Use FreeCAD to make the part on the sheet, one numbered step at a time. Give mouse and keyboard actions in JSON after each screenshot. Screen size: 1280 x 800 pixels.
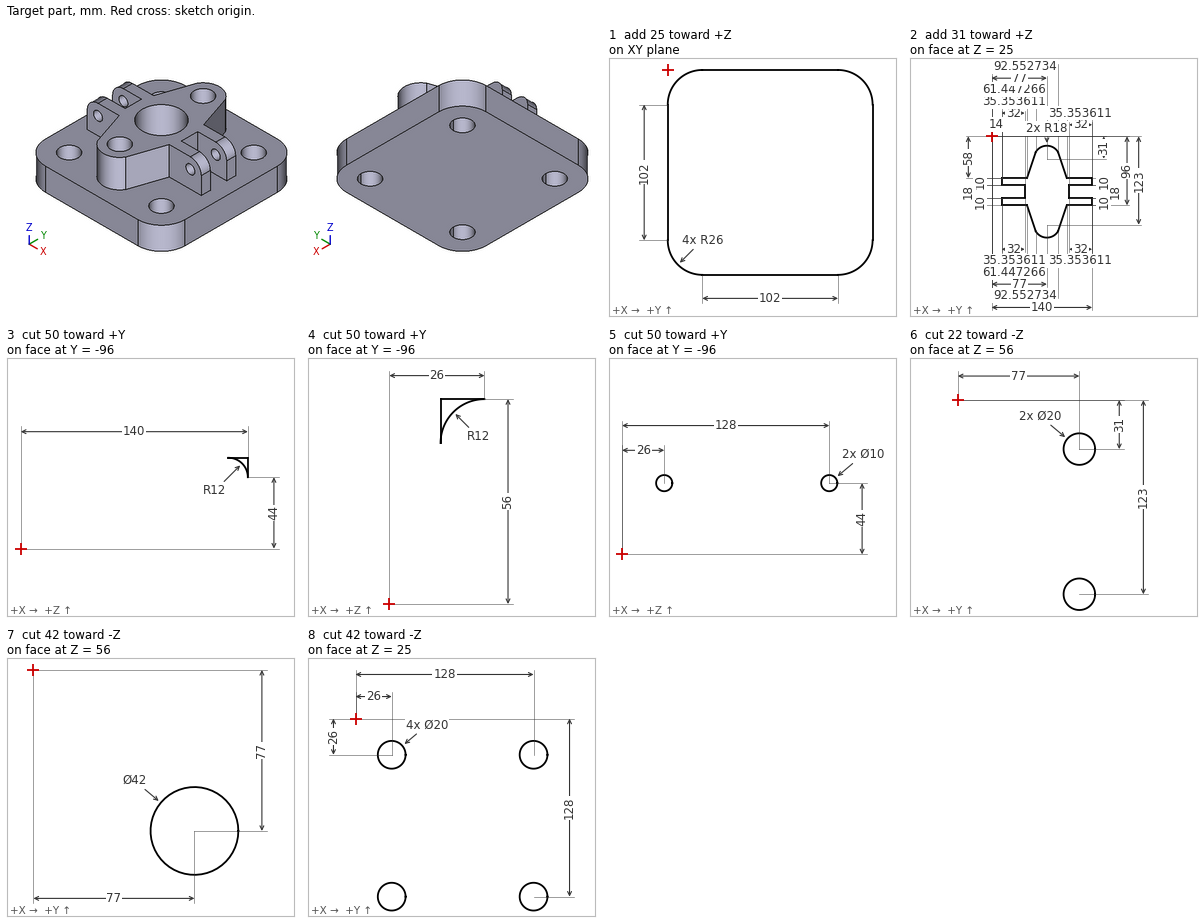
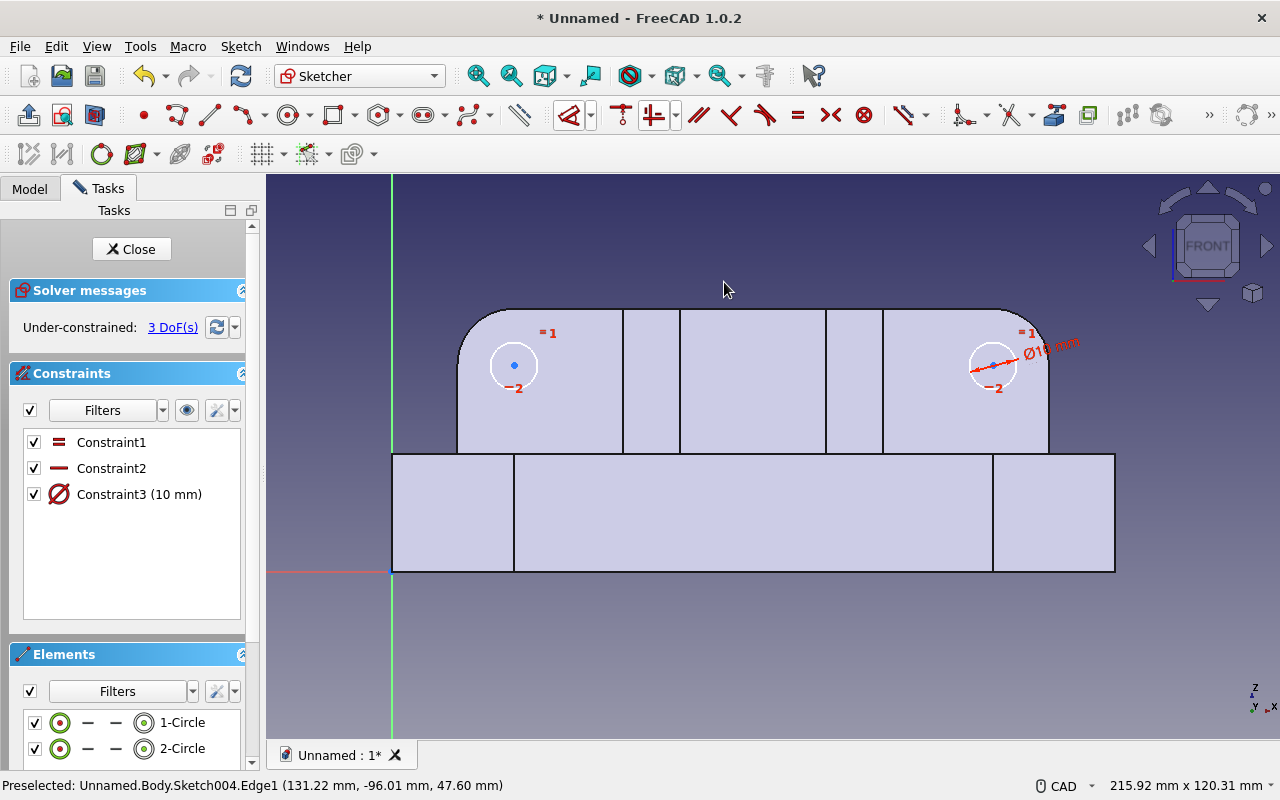
{"action": "left_click", "coordinate": [993, 366]}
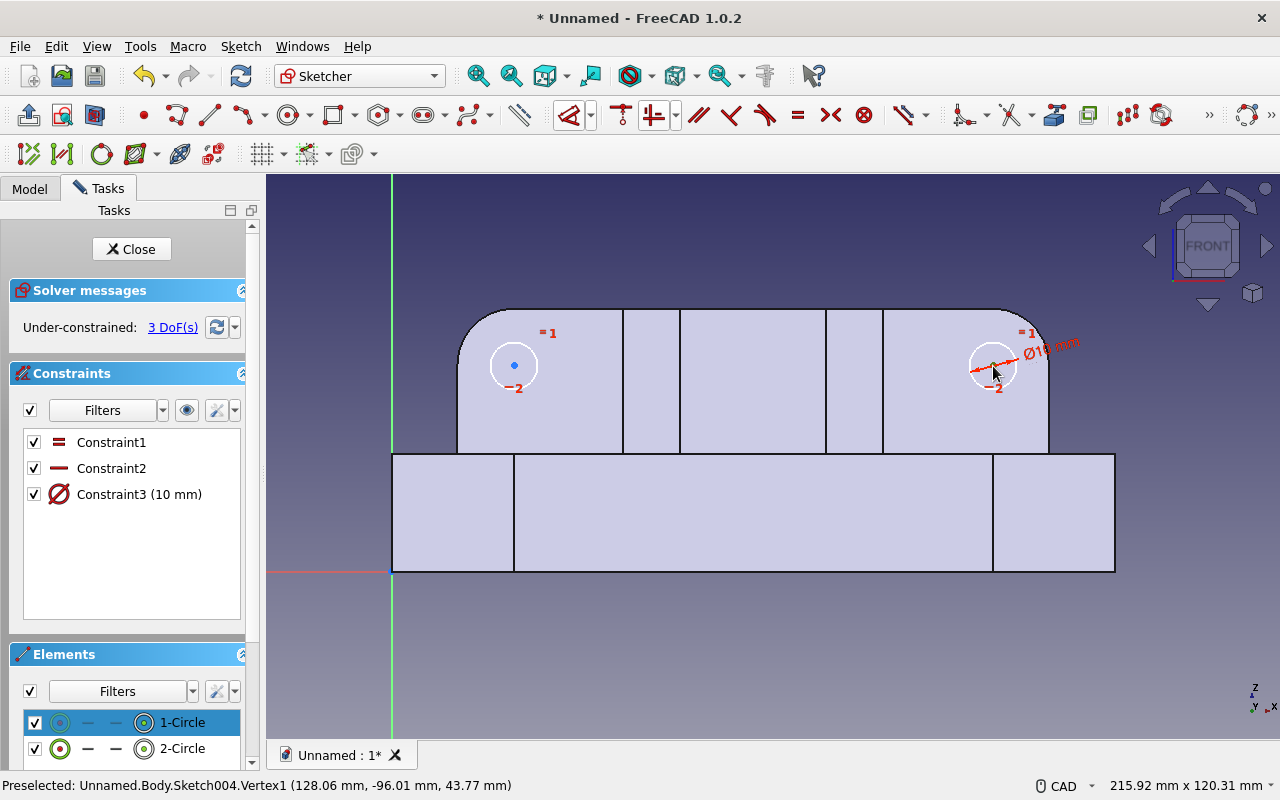
{"action": "left_click", "coordinate": [590, 116]}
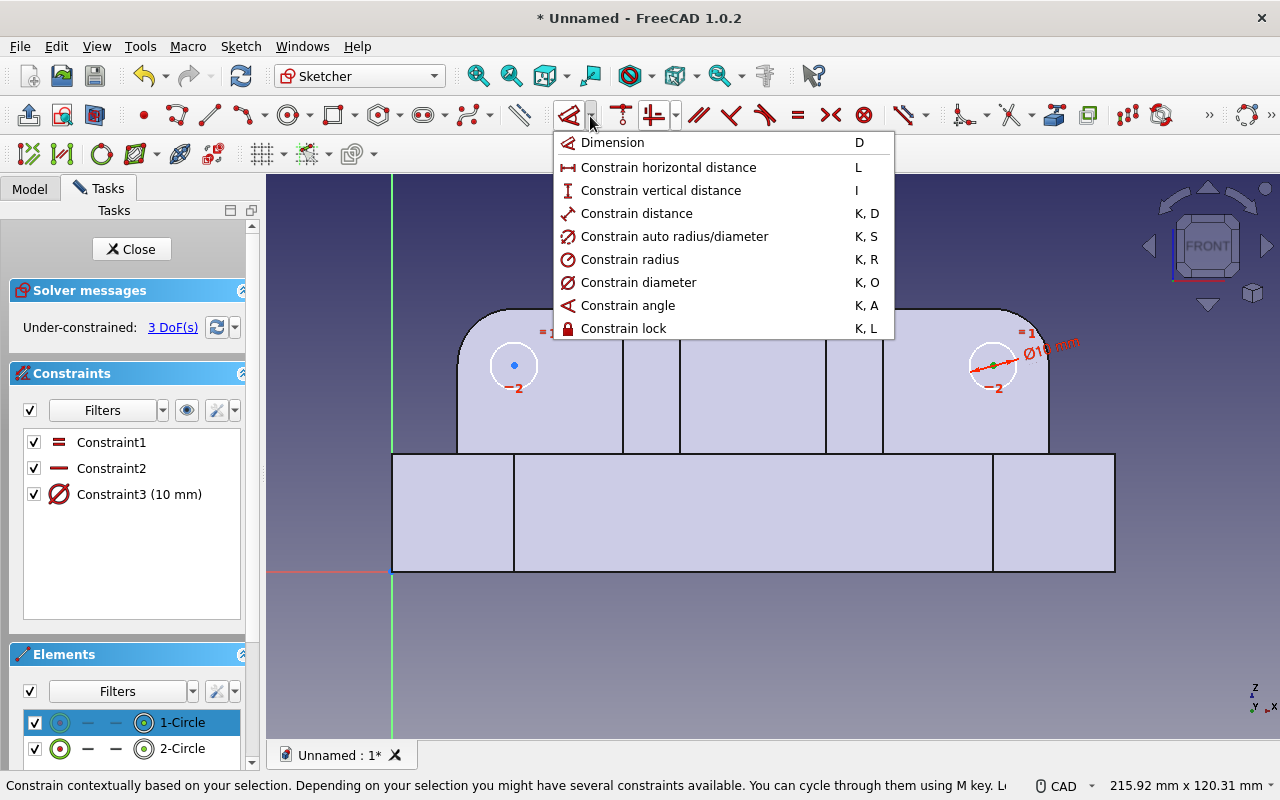
{"action": "left_click", "coordinate": [724, 190]}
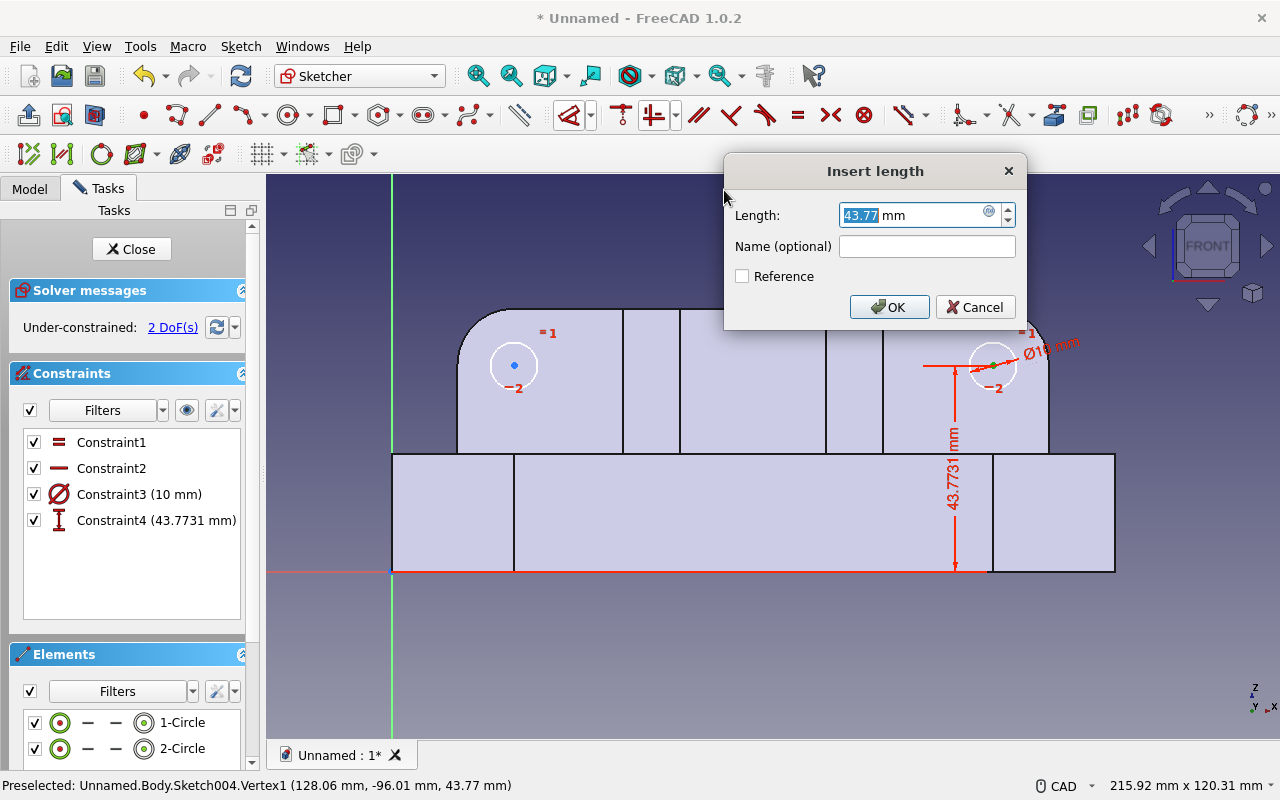
{"action": "type", "text": "44"}
{"action": "key", "text": "Return"}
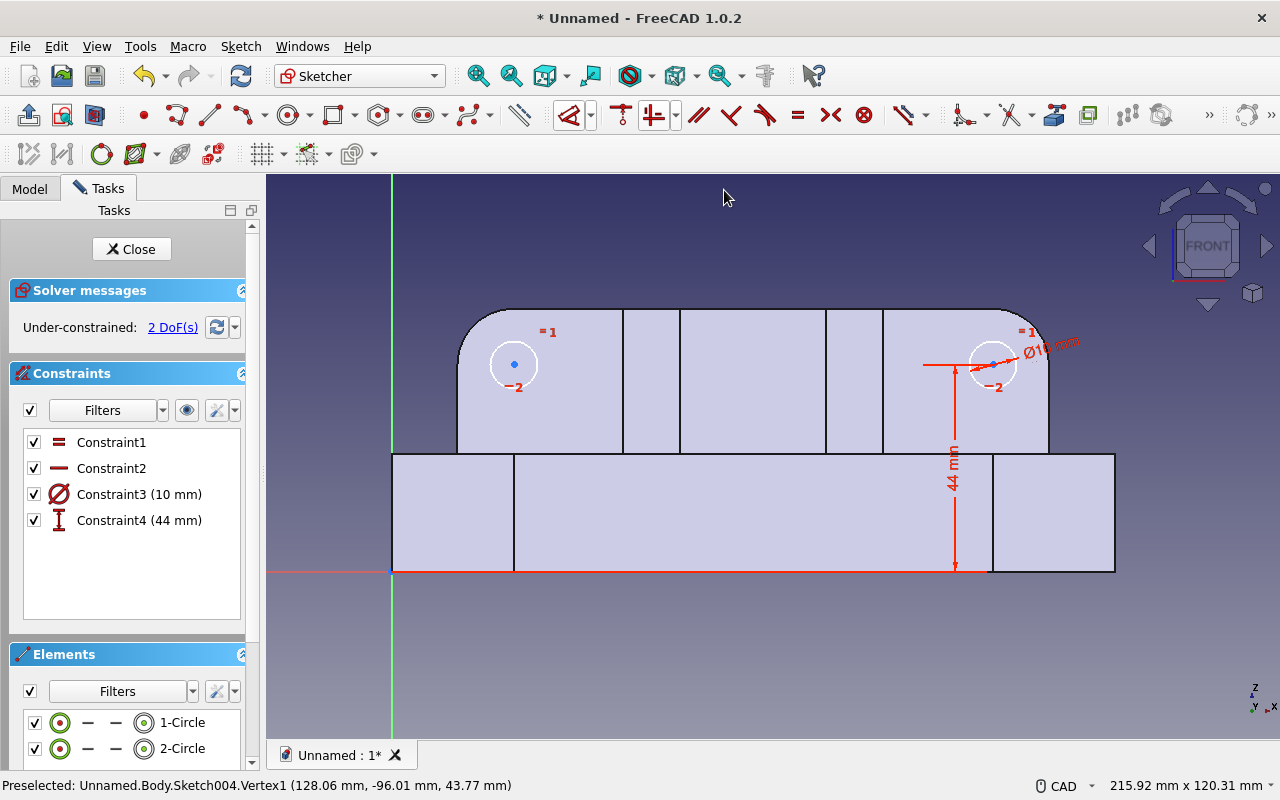
{"action": "left_click", "coordinate": [514, 365]}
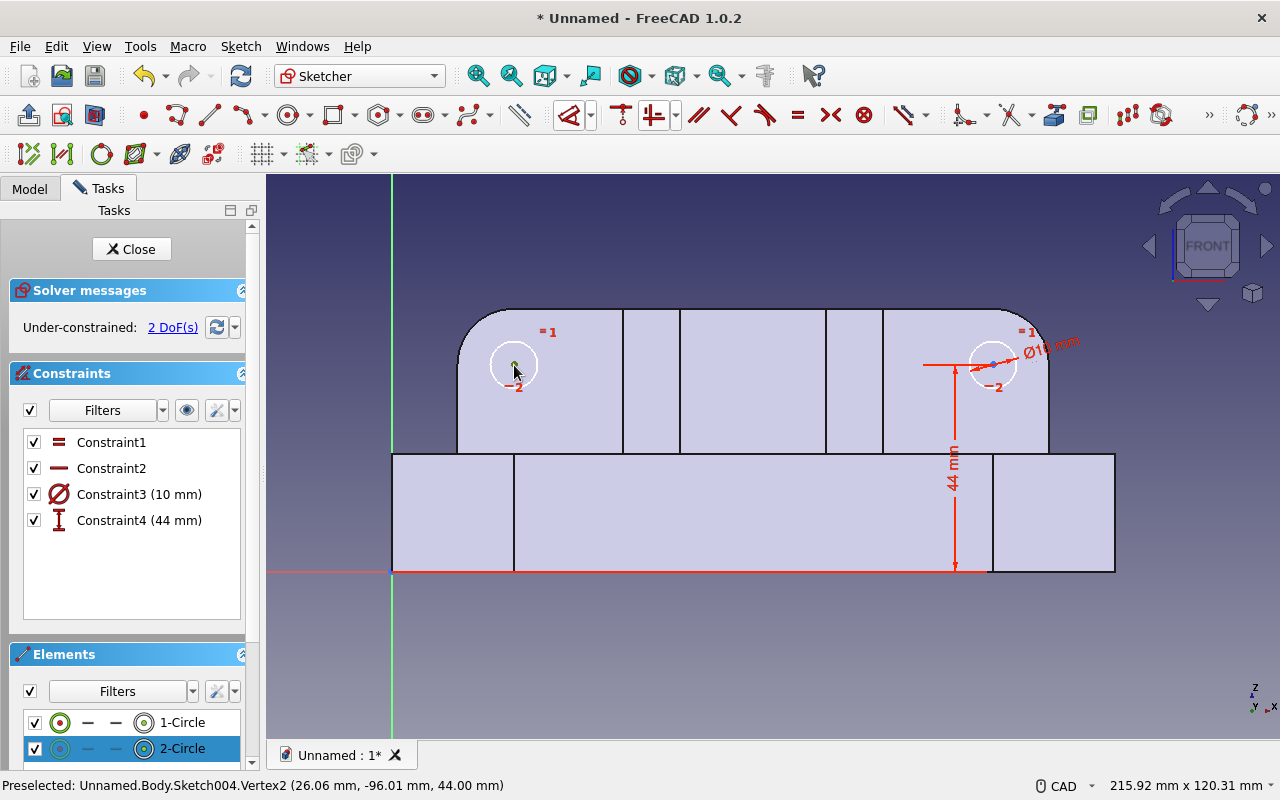
{"action": "key", "text": "l"}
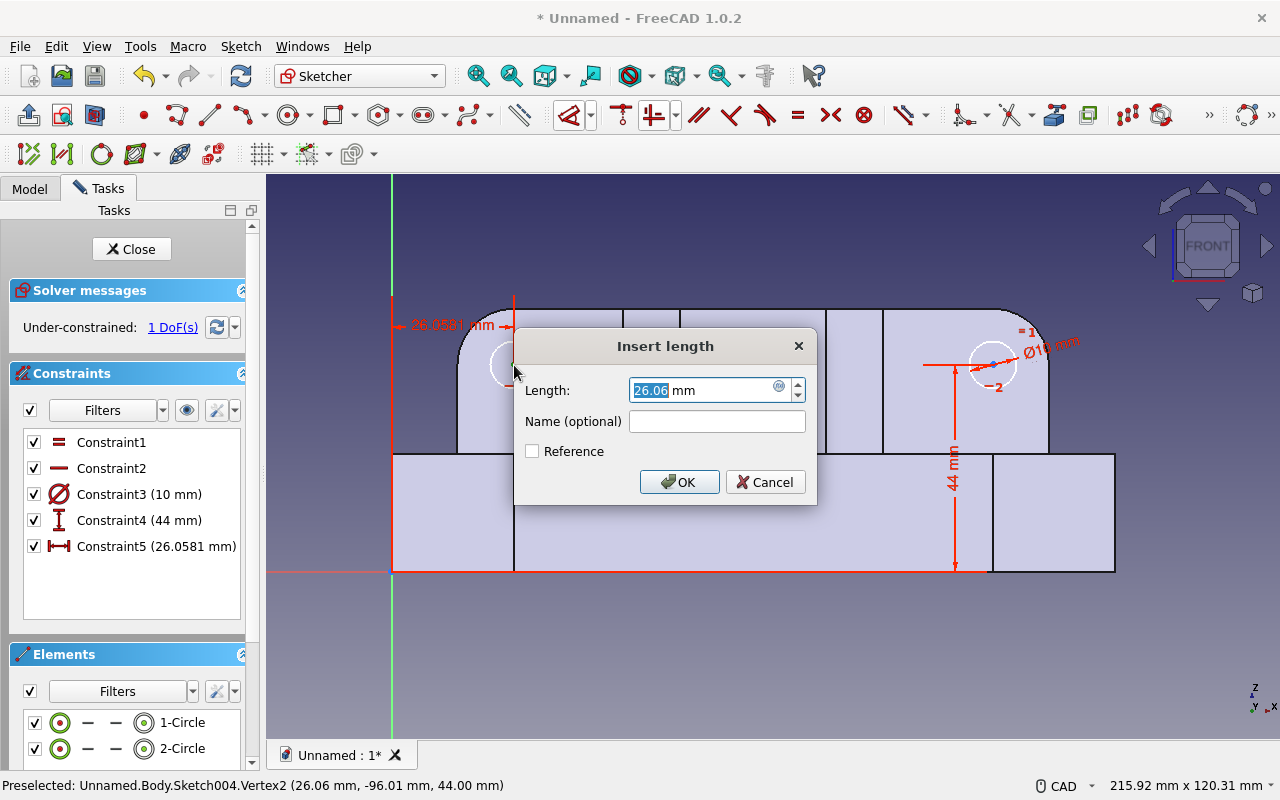
{"action": "type", "text": "26"}
{"action": "key", "text": "Return"}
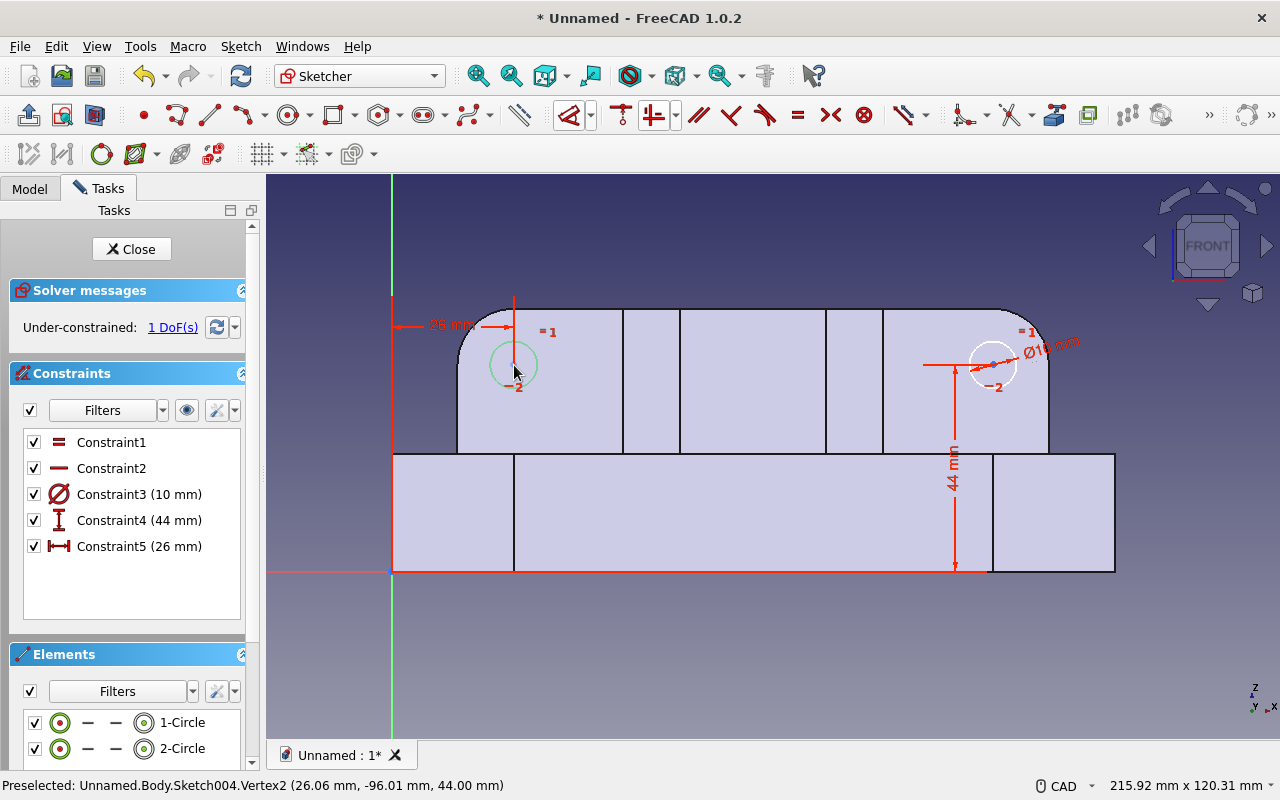
{"action": "left_click", "coordinate": [993, 365]}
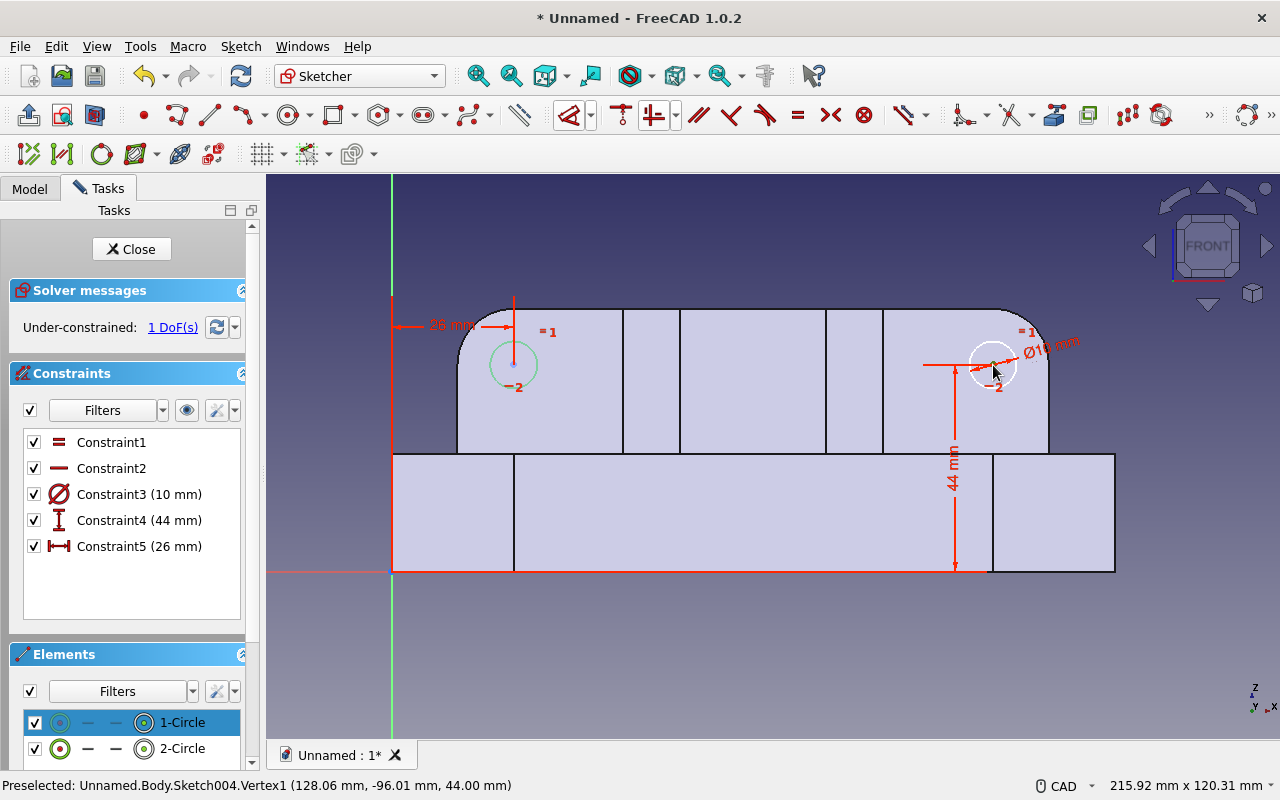
{"action": "left_click", "coordinate": [590, 116]}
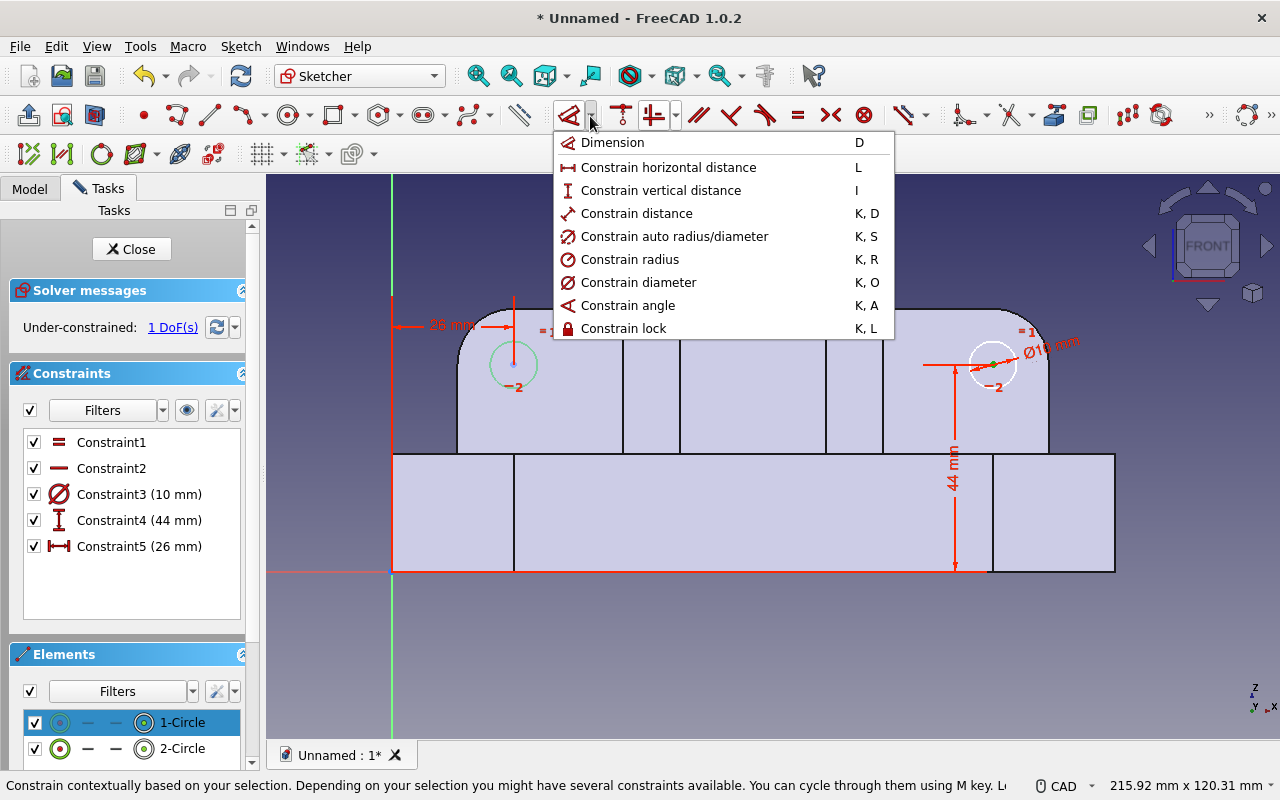
{"action": "left_click", "coordinate": [724, 168]}